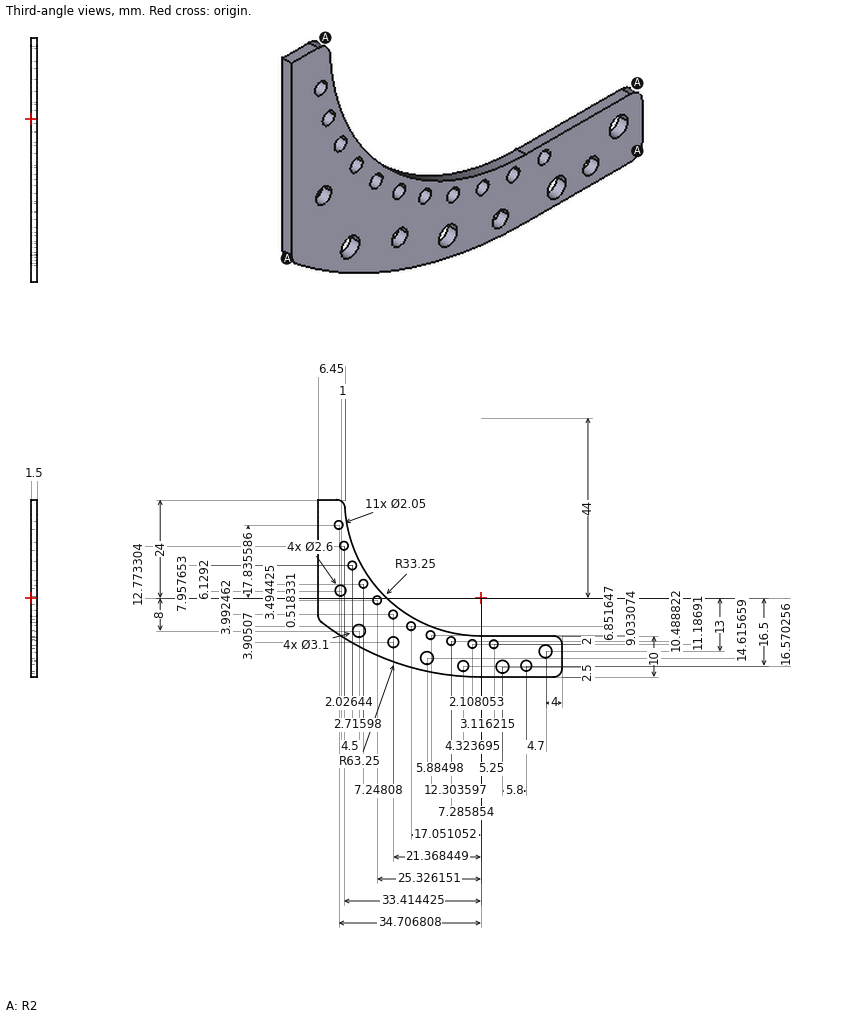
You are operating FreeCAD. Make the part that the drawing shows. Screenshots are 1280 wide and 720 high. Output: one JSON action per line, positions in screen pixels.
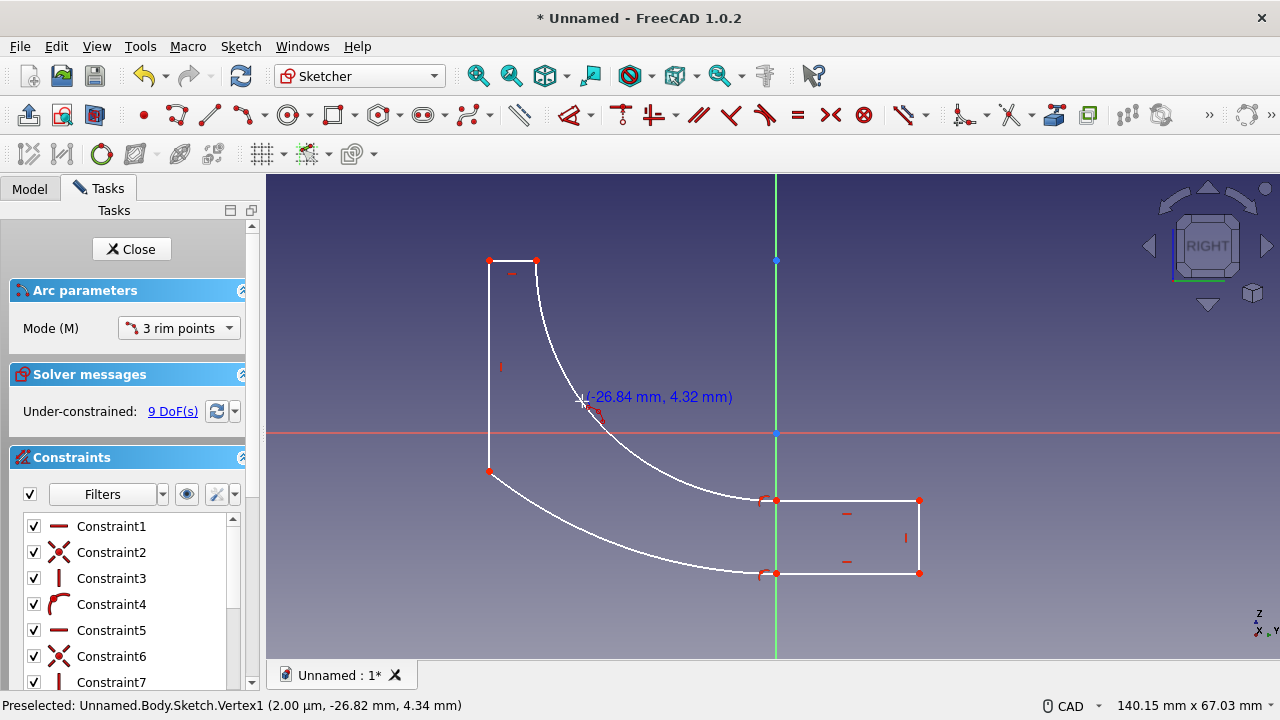
{"action": "left_click", "coordinate": [288, 116]}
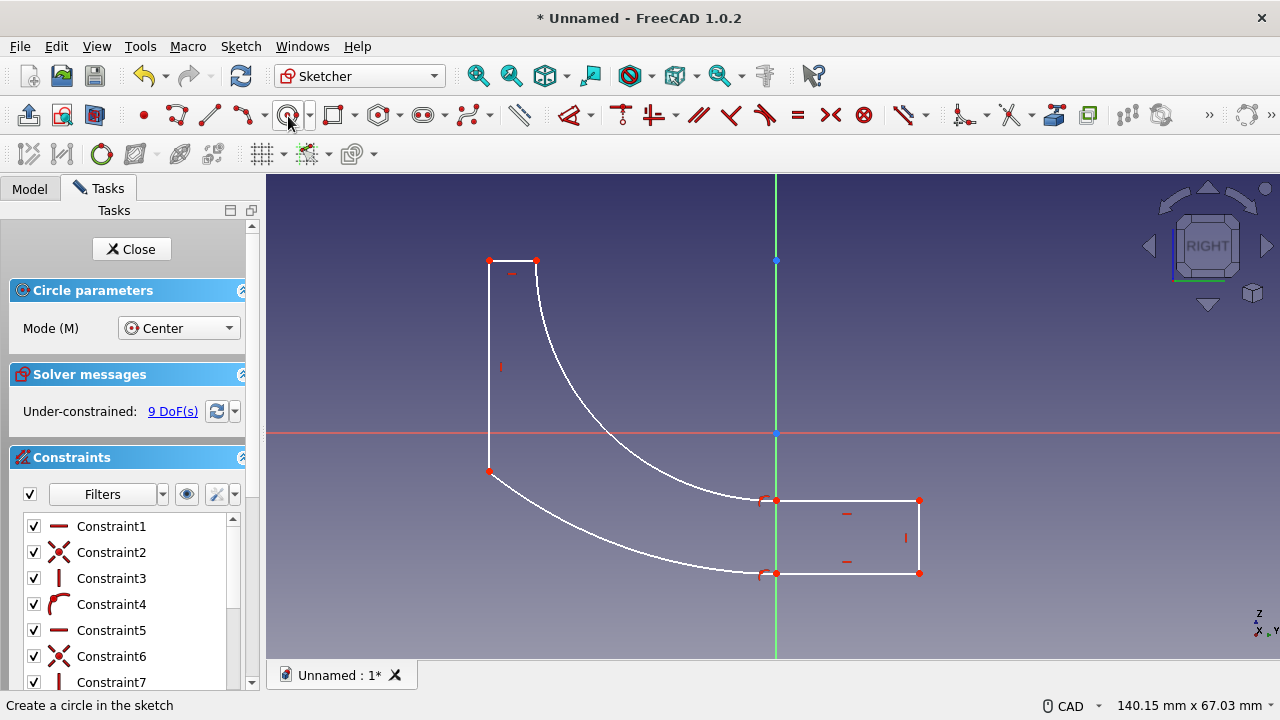
{"action": "scroll", "coordinate": [525, 304], "scroll_direction": "up", "scroll_amount": 6}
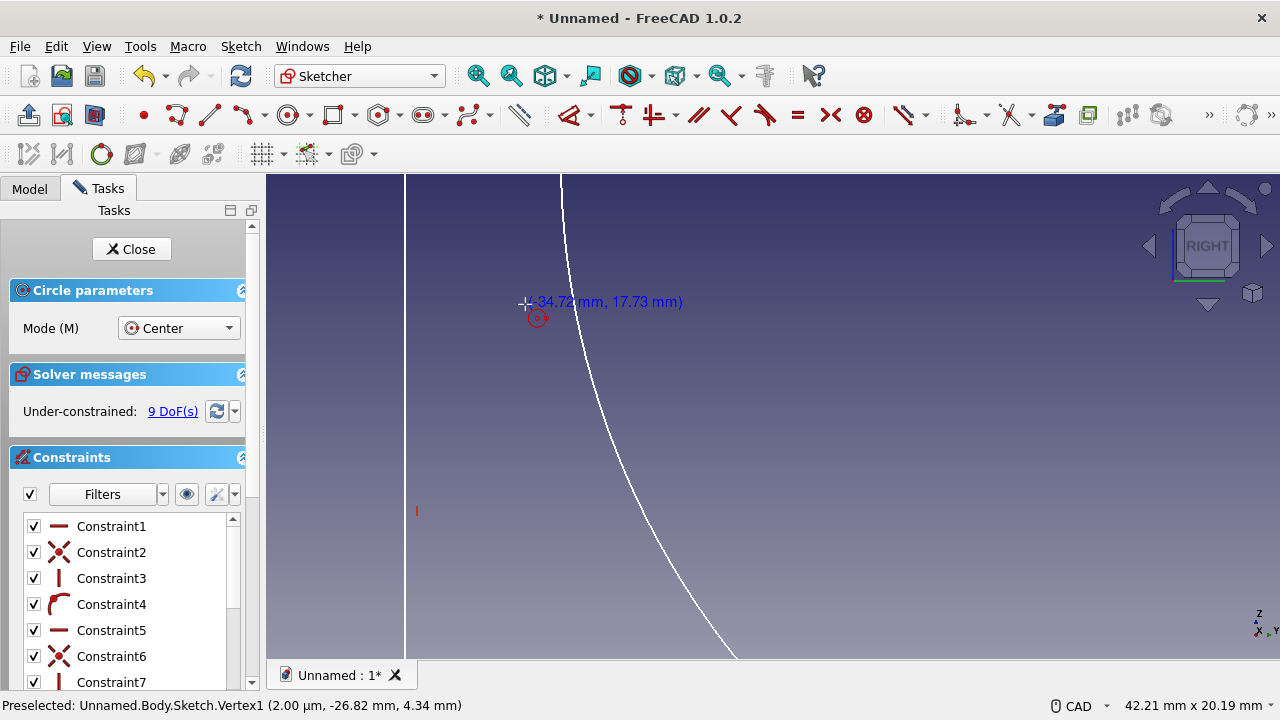
{"action": "left_click", "coordinate": [525, 304]}
{"action": "mouse_move", "coordinate": [542, 287]}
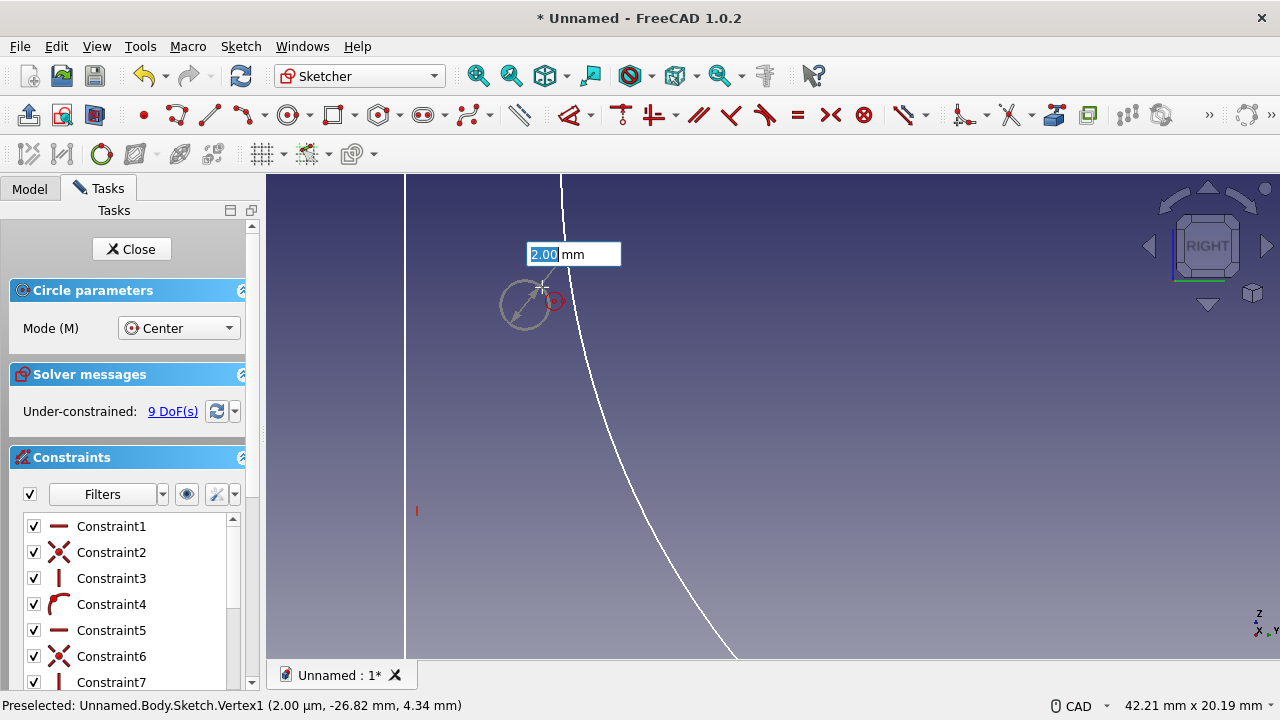
{"action": "type", "text": "2.05"}
{"action": "key", "text": "Return"}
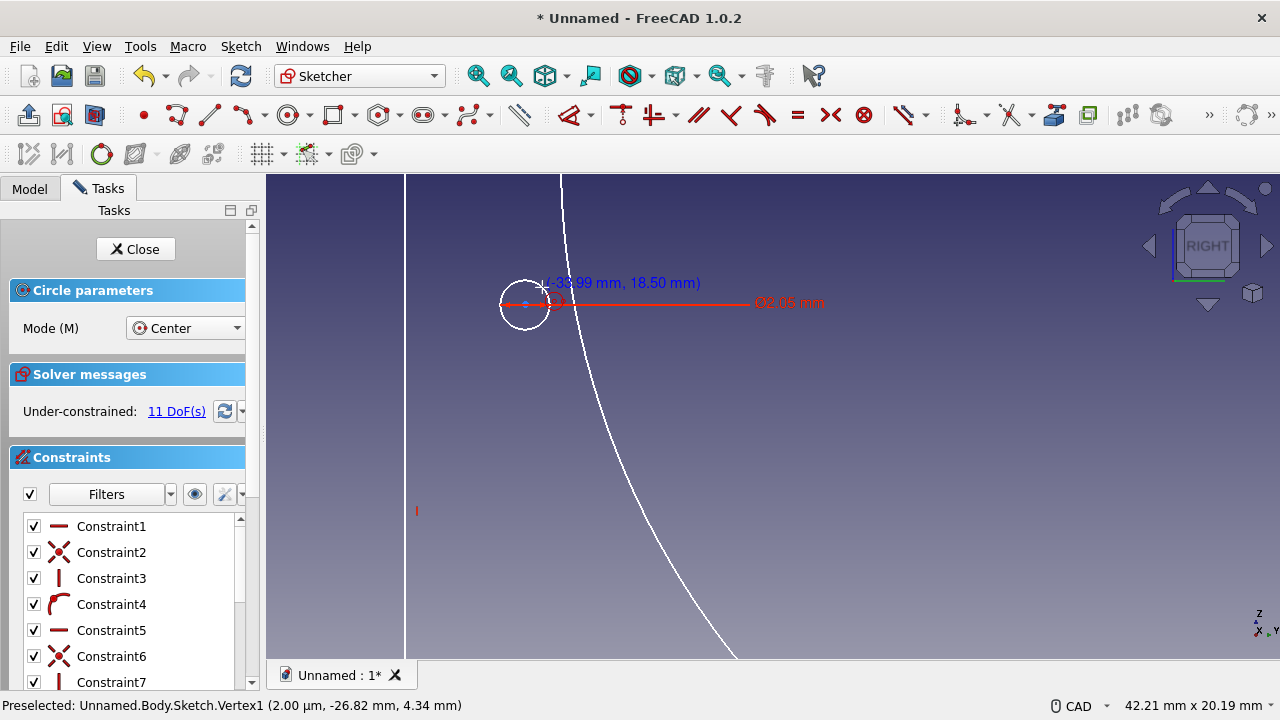
{"action": "left_click", "coordinate": [556, 426]}
{"action": "mouse_move", "coordinate": [573, 408]}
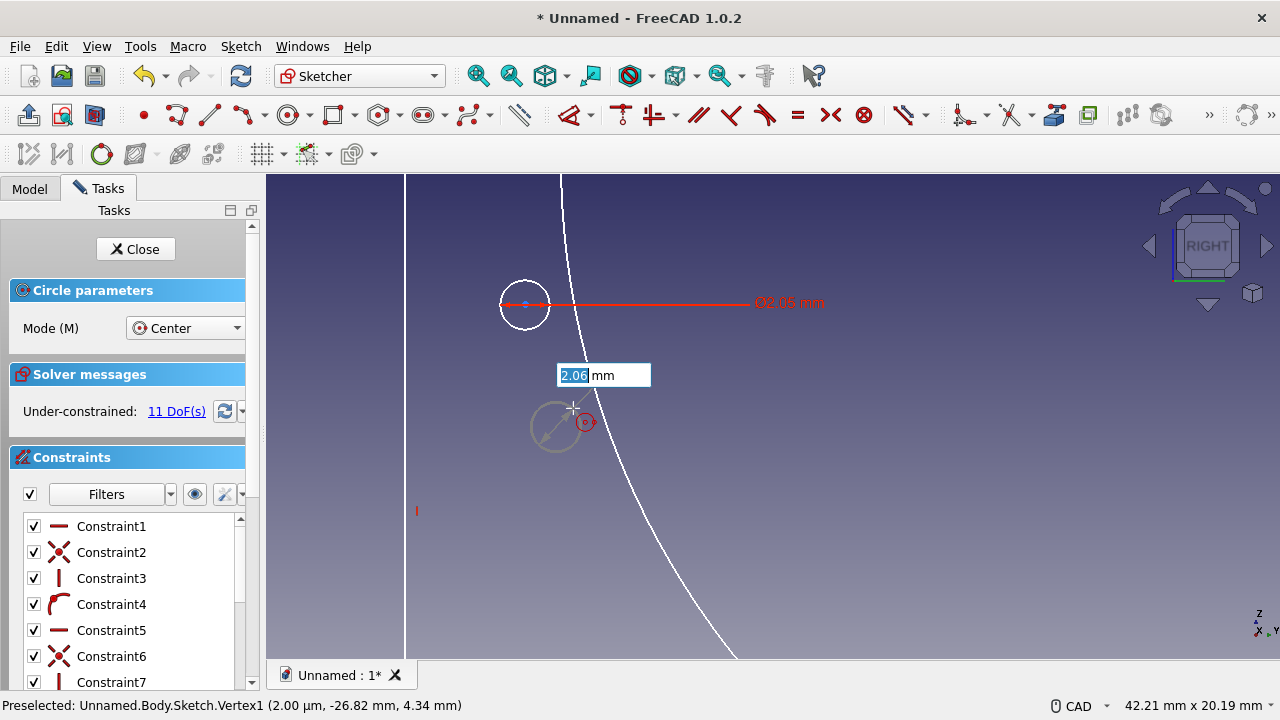
{"action": "type", "text": "2.05"}
{"action": "key", "text": "Return"}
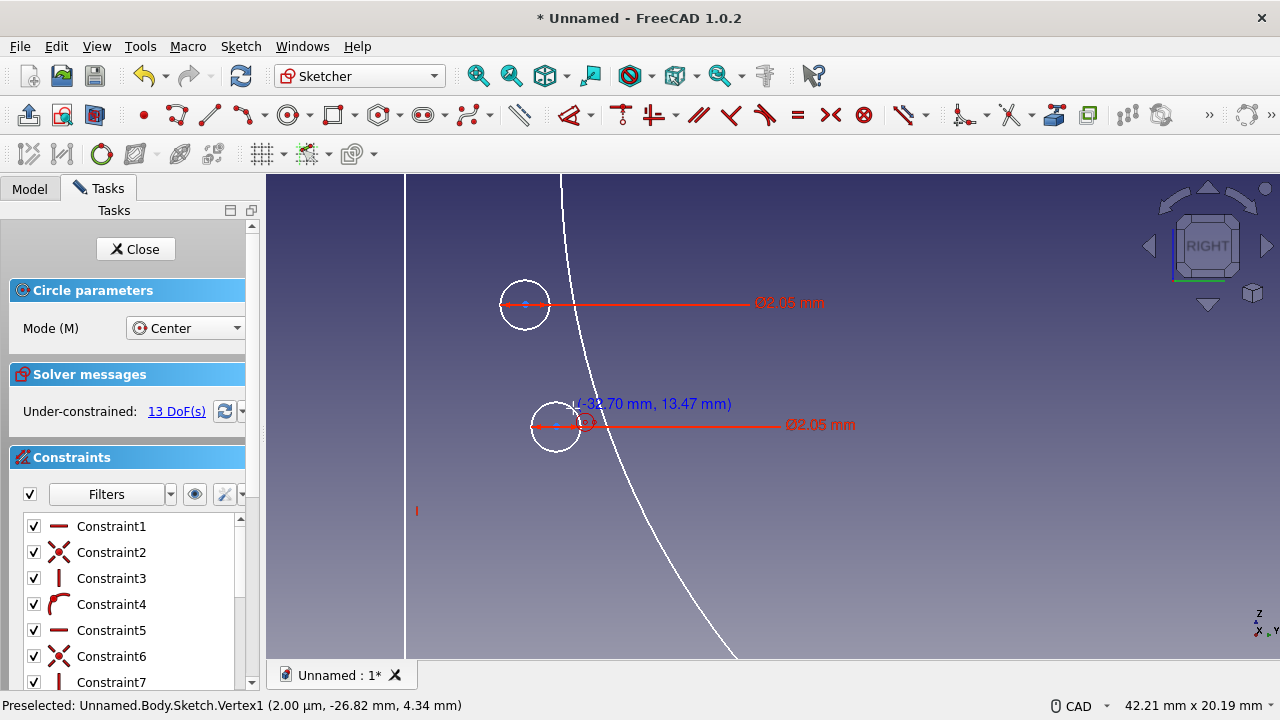
{"action": "left_click", "coordinate": [604, 541]}
{"action": "mouse_move", "coordinate": [622, 524]}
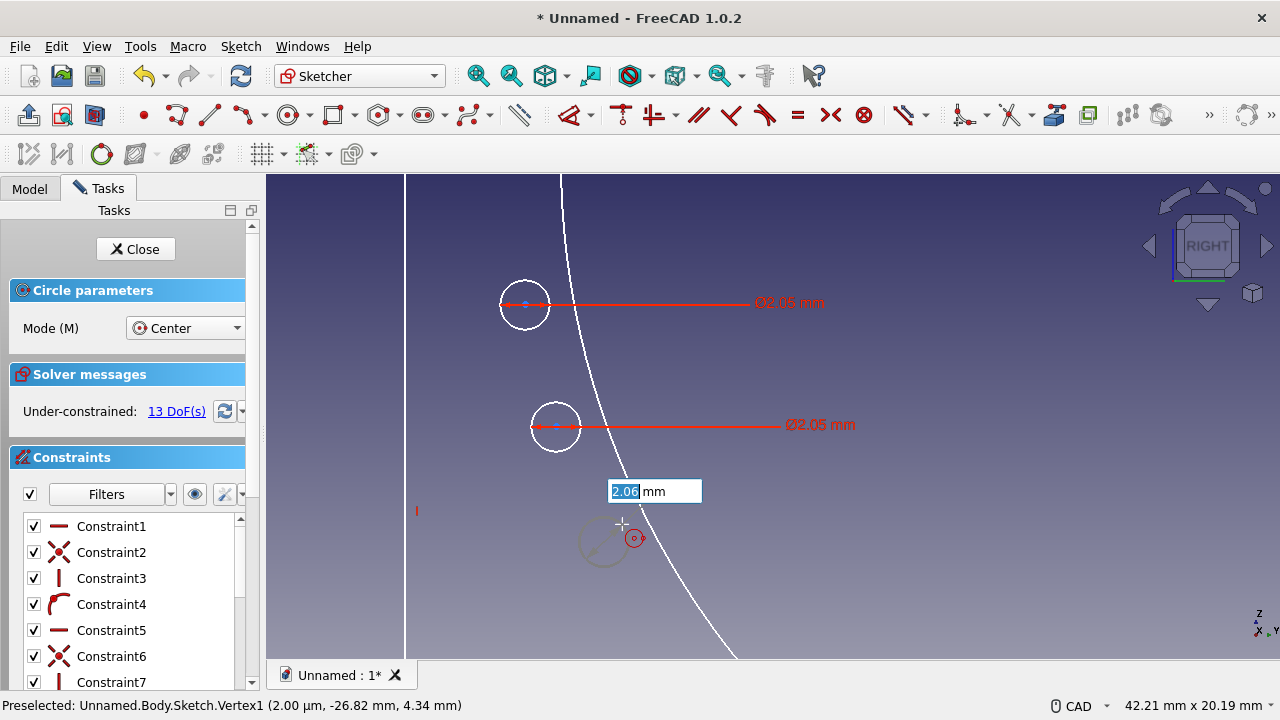
{"action": "type", "text": "2.05"}
{"action": "key", "text": "Return"}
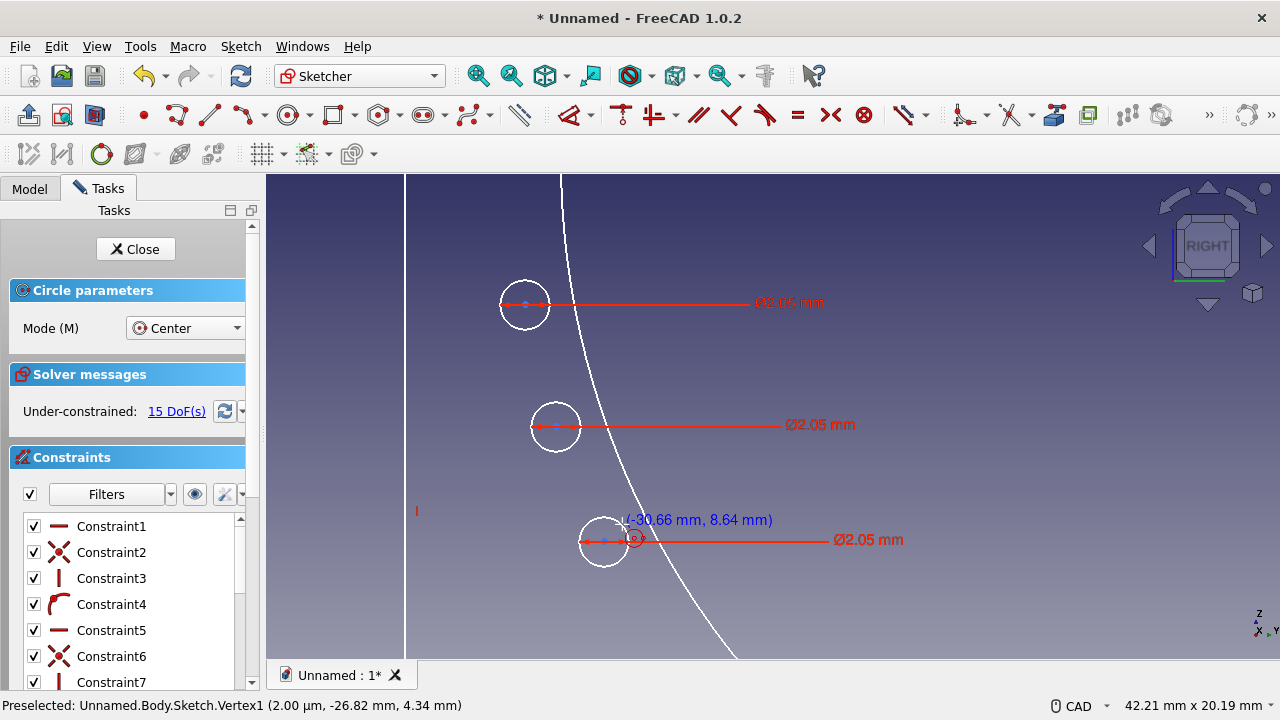
{"action": "scroll", "coordinate": [526, 305], "scroll_direction": "down", "scroll_amount": 6}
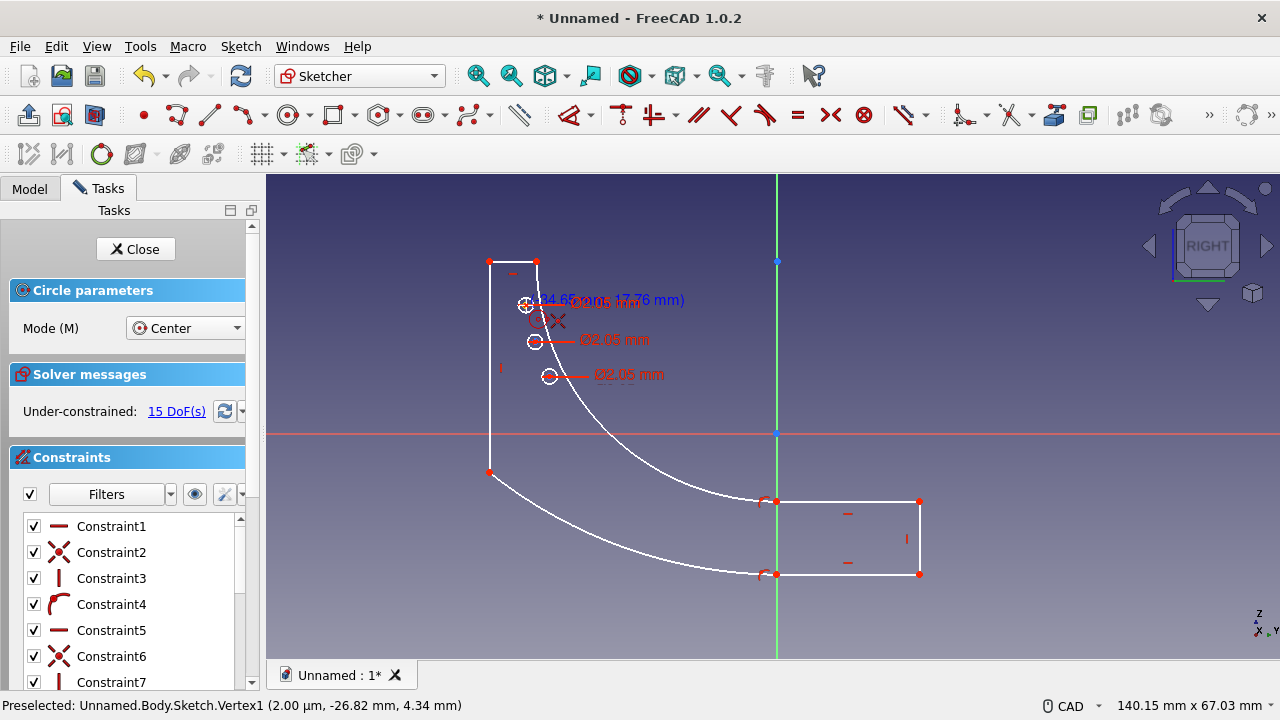
{"action": "scroll", "coordinate": [529, 421], "scroll_direction": "up", "scroll_amount": 5}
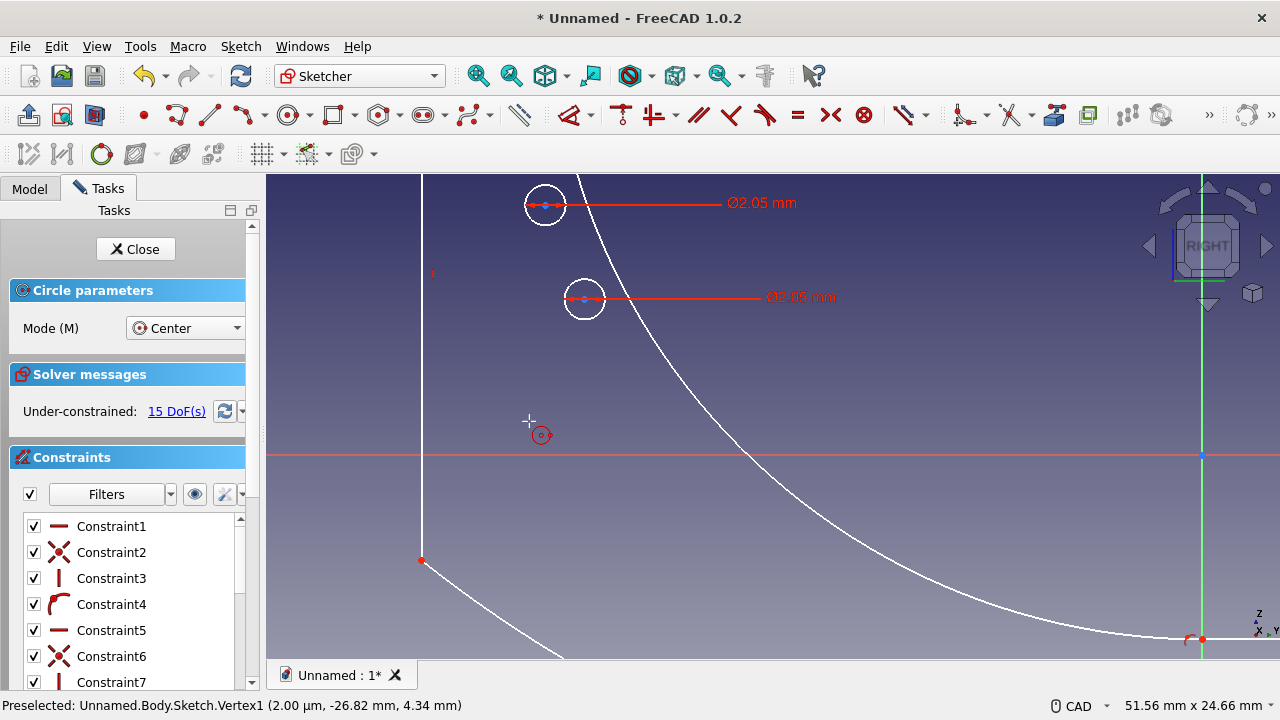
{"action": "left_click", "coordinate": [529, 419]}
{"action": "mouse_move", "coordinate": [547, 401]}